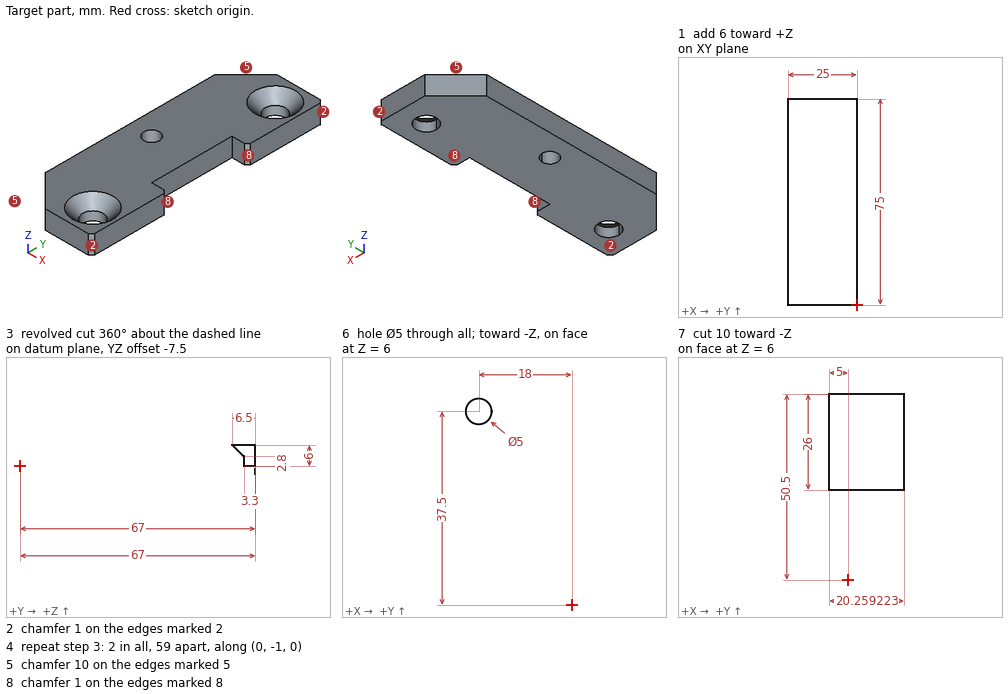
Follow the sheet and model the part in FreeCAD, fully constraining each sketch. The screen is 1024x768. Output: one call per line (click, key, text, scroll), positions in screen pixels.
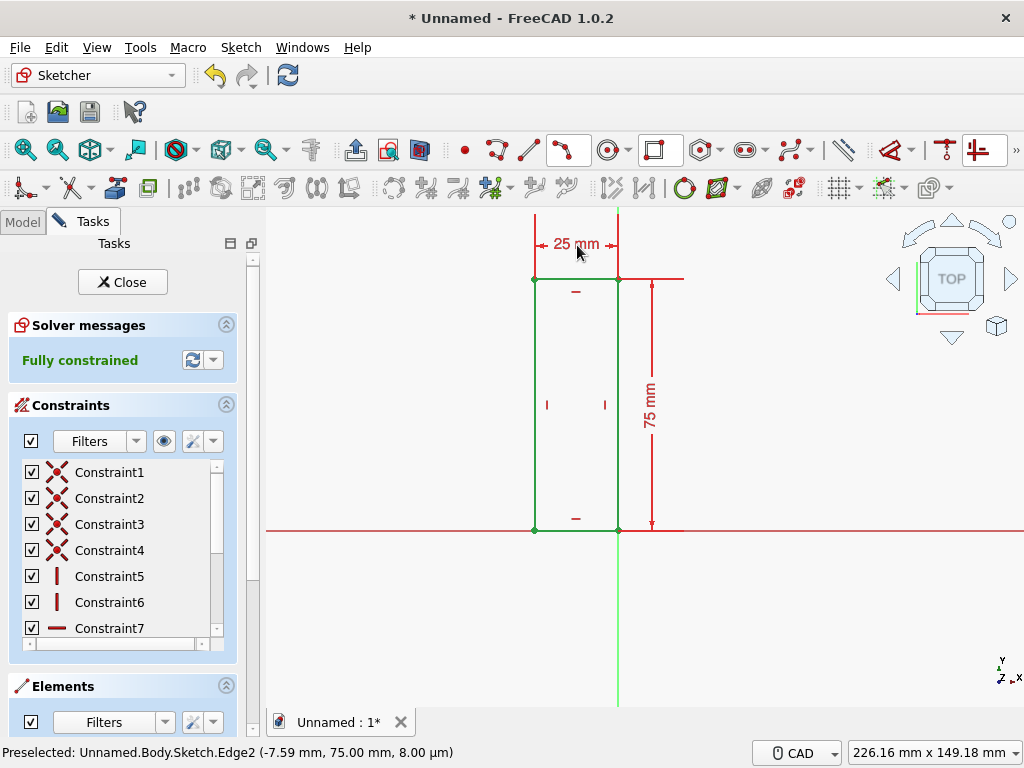
click(123, 282)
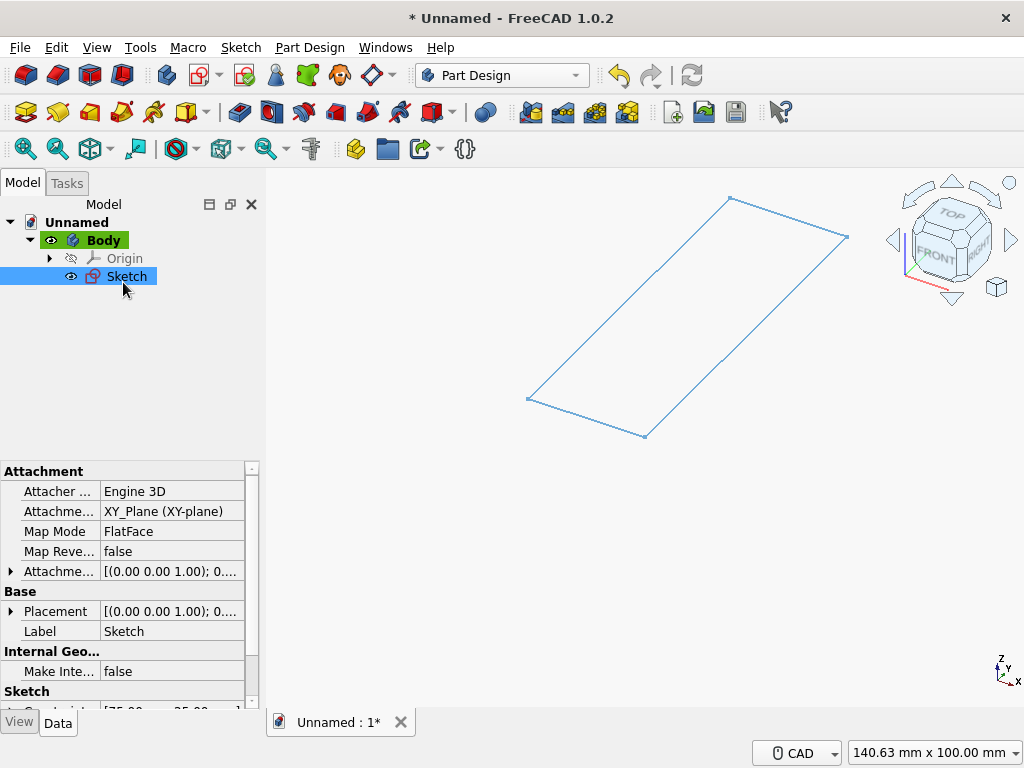
click(26, 112)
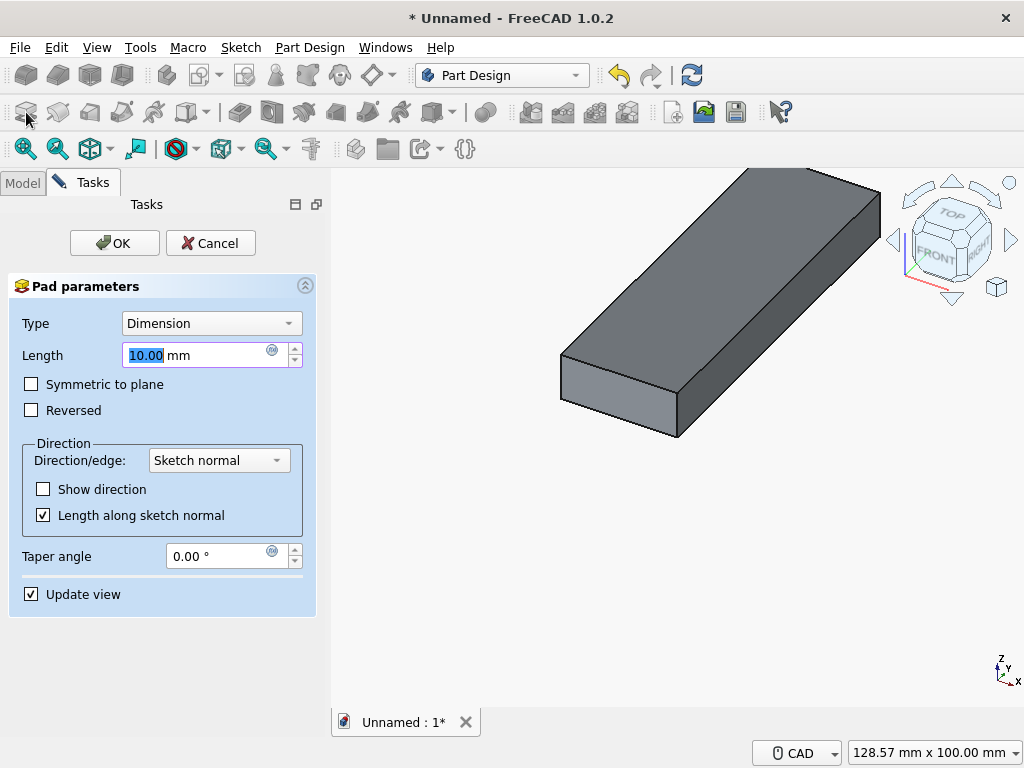
text(6)
key(Tab)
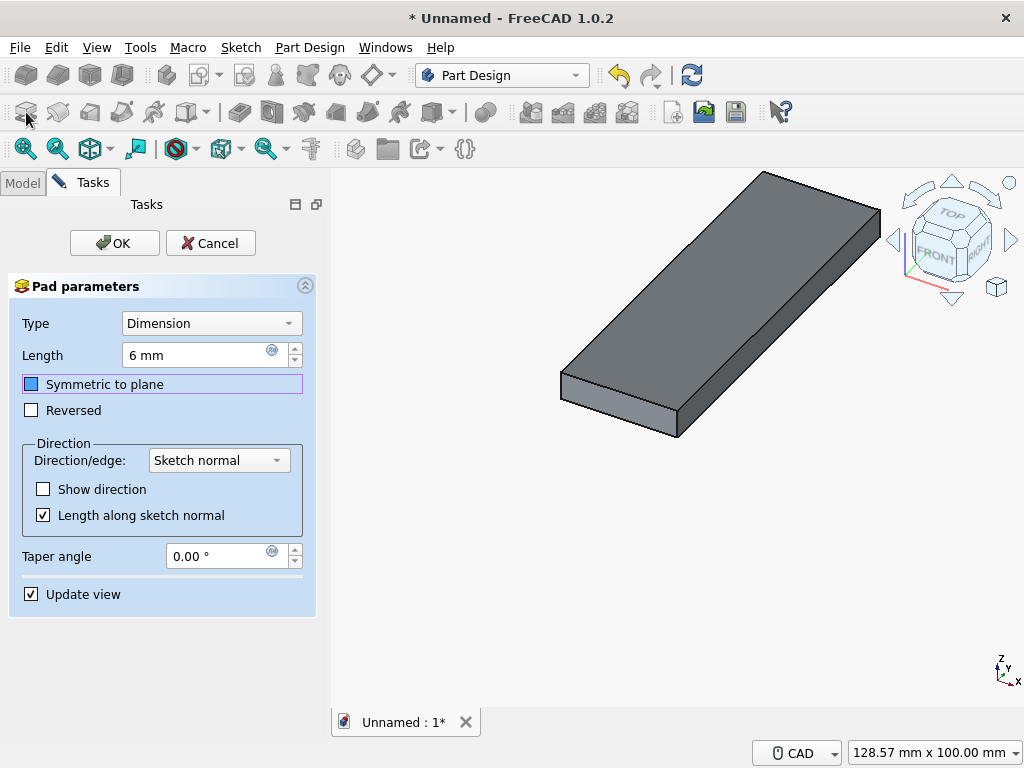
click(115, 243)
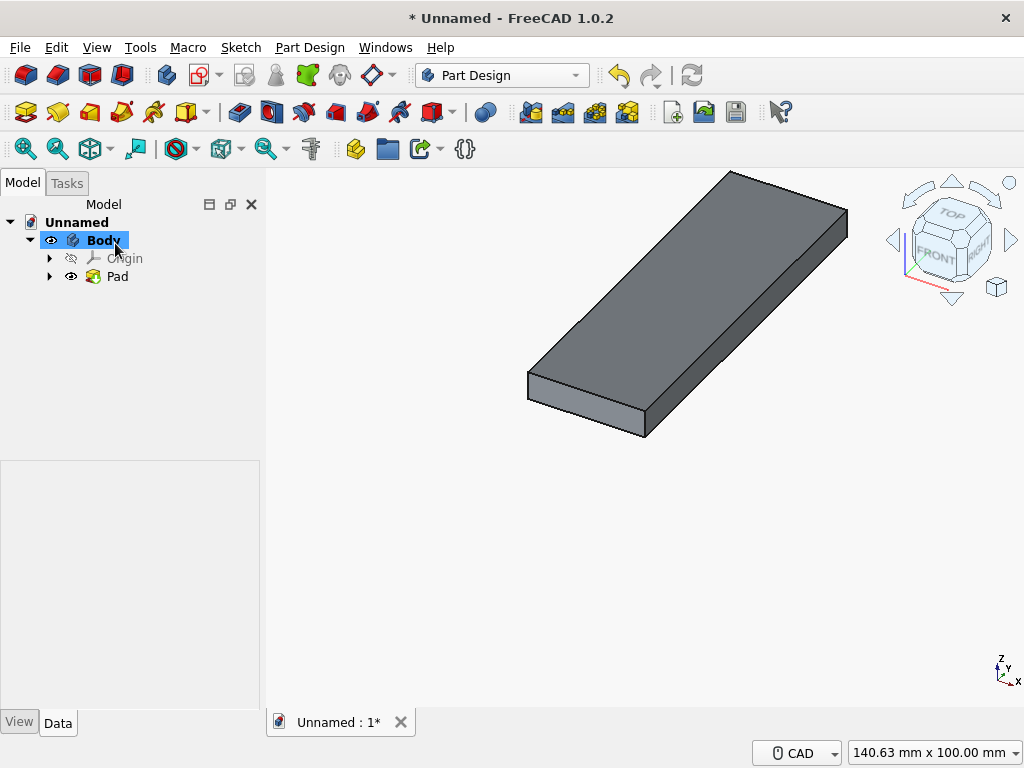
click(645, 423)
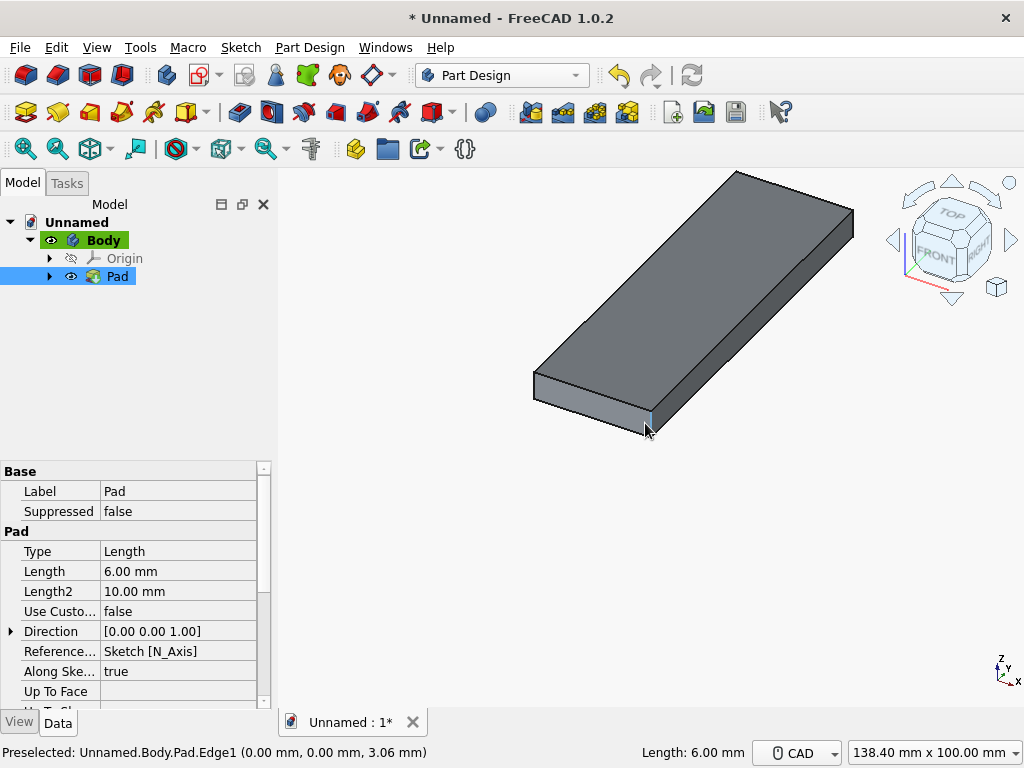
key(0)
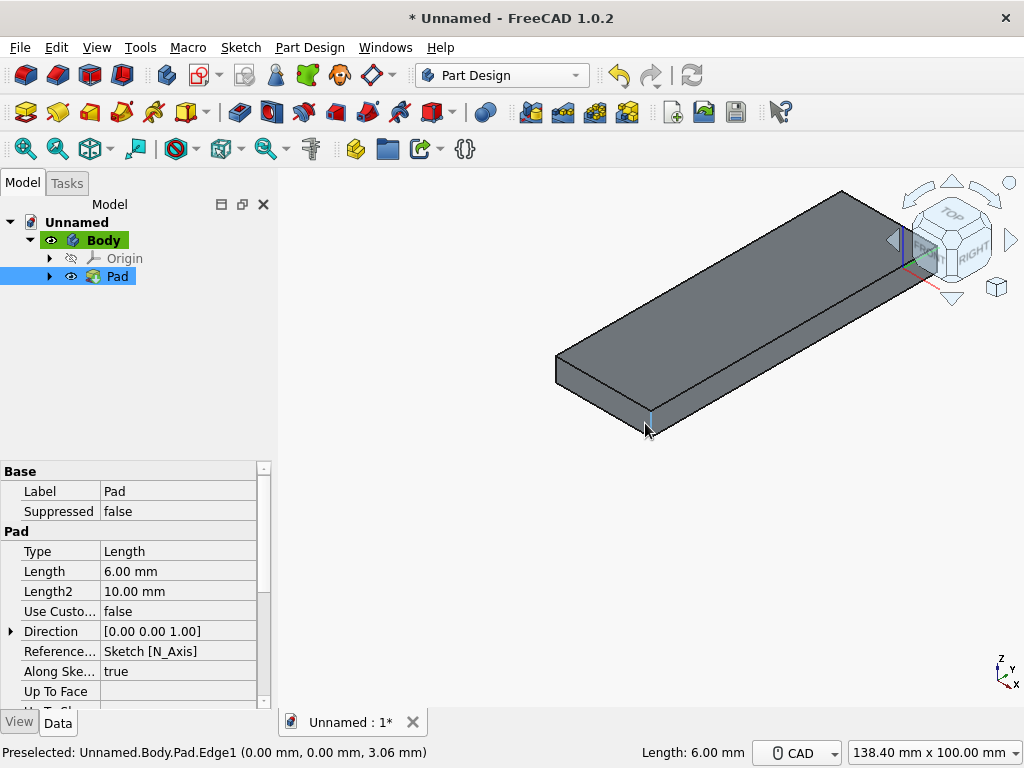
key(2)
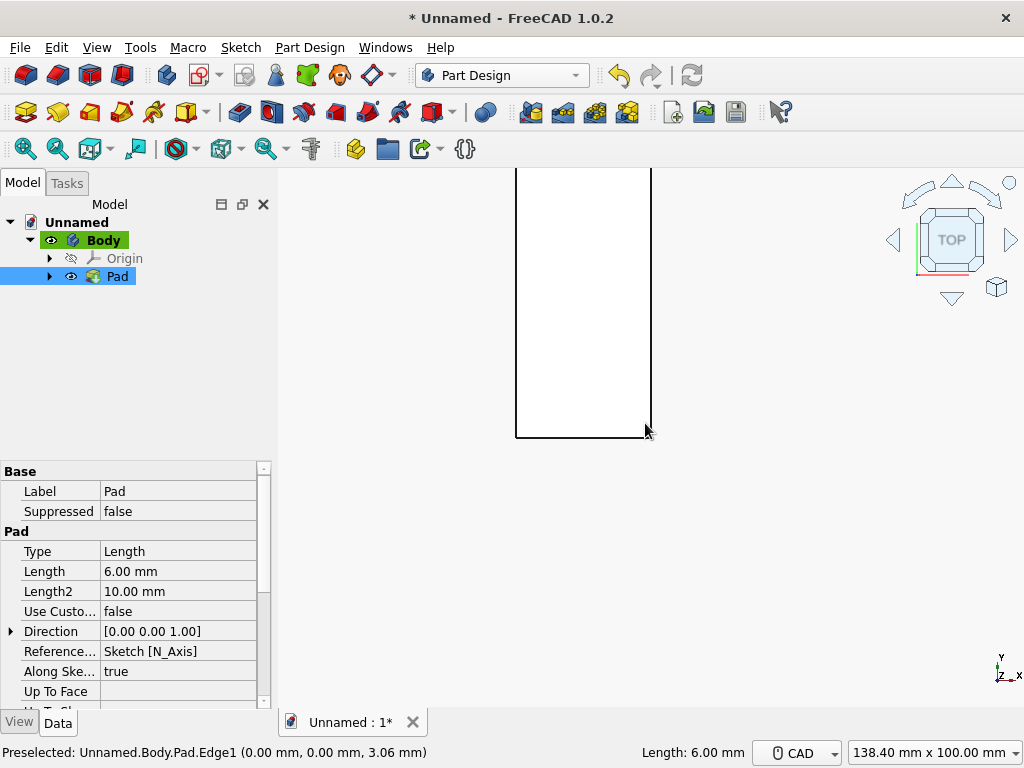
click(26, 150)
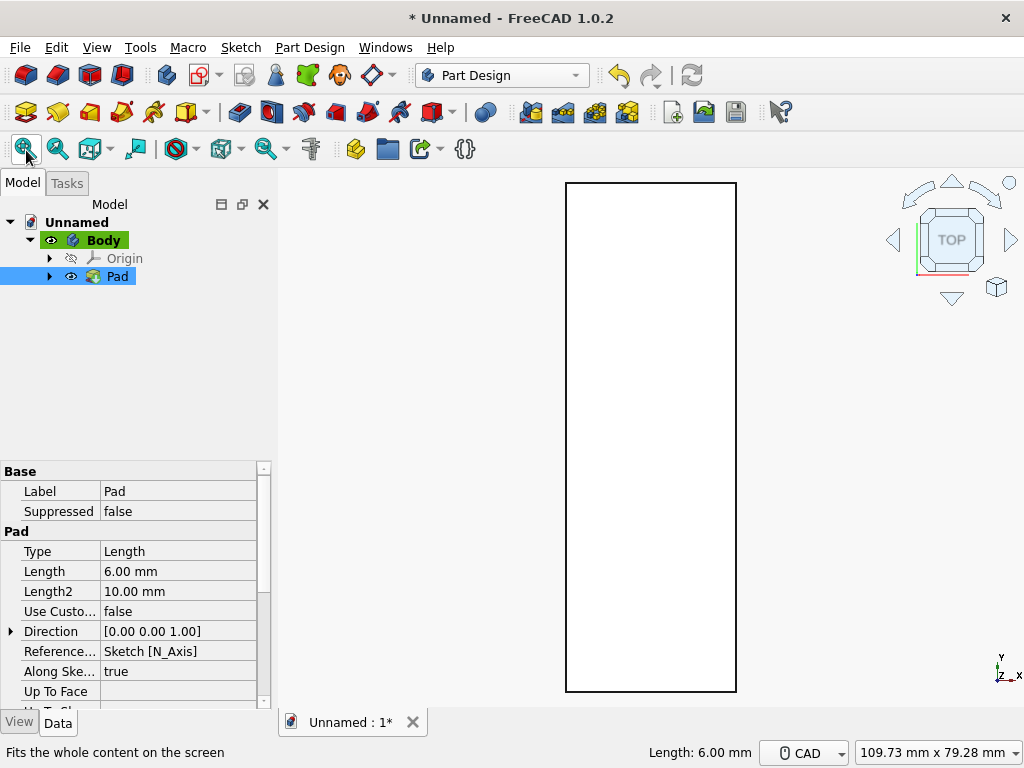
key(1)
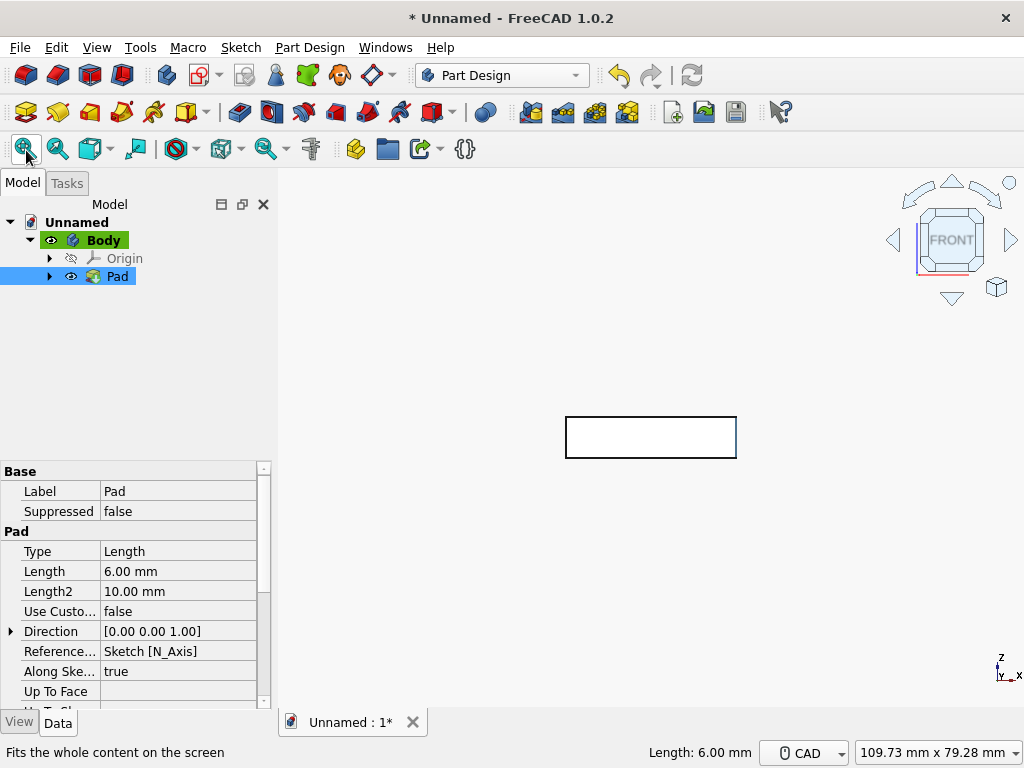
click(26, 150)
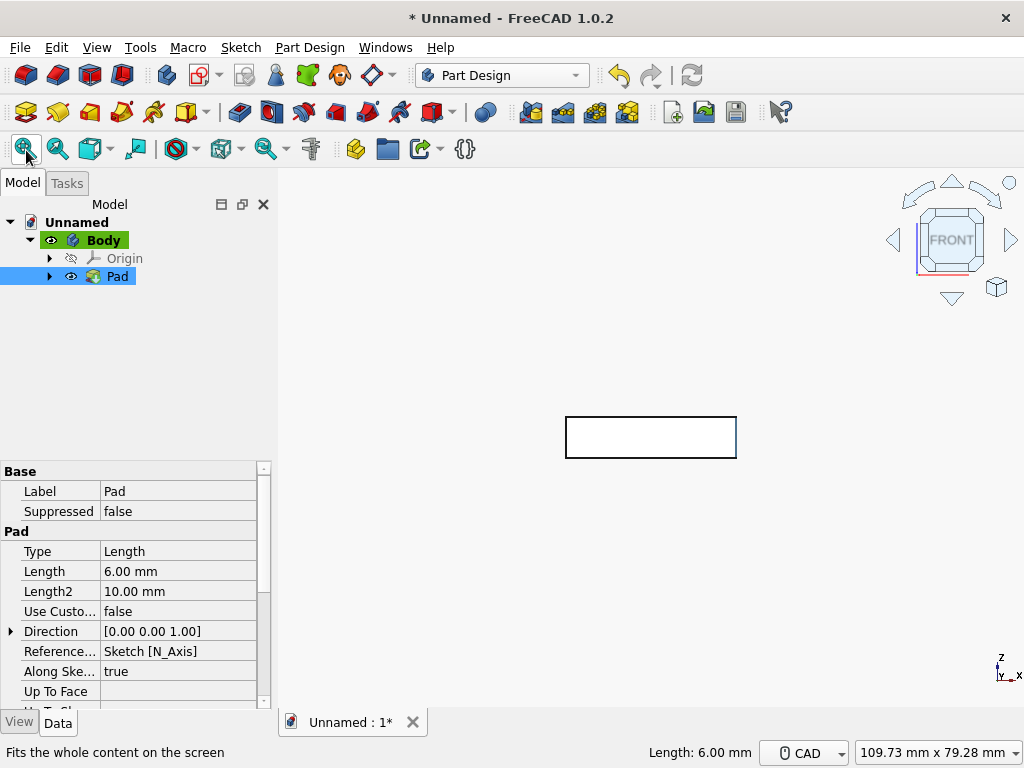
key(3)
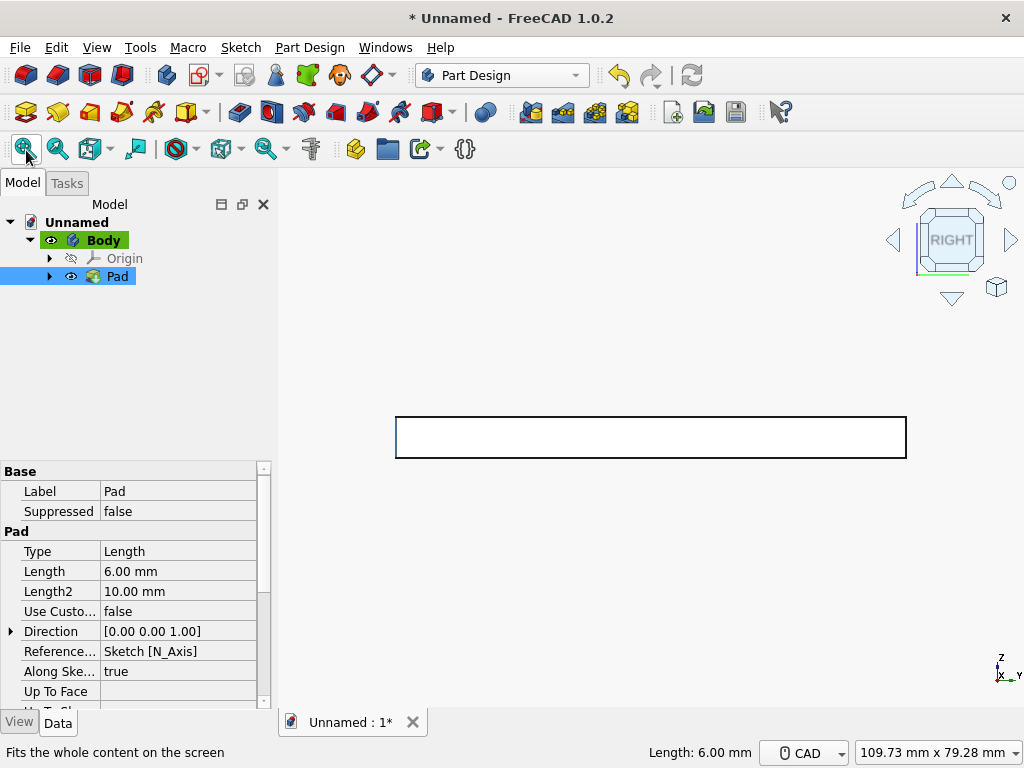
click(906, 436, ctrl)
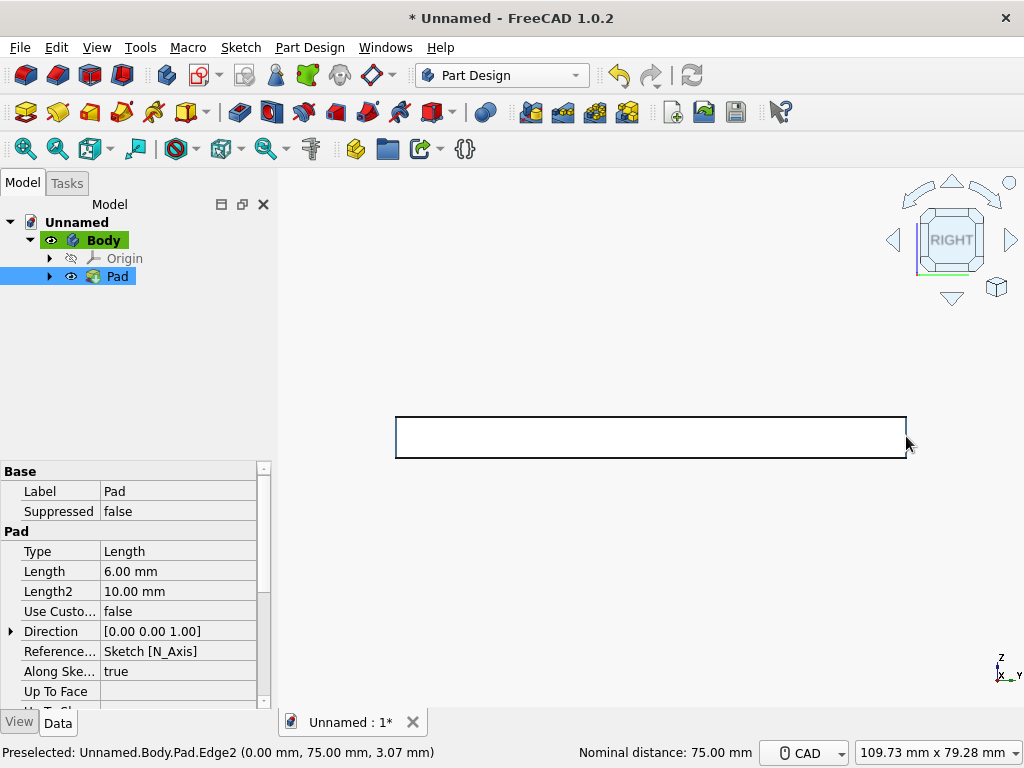
click(58, 76)